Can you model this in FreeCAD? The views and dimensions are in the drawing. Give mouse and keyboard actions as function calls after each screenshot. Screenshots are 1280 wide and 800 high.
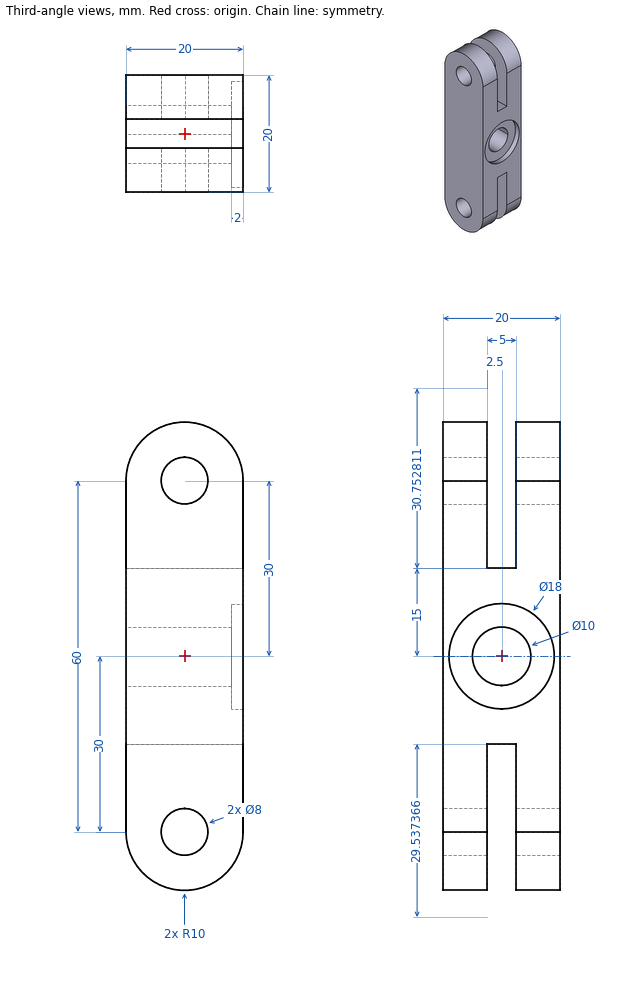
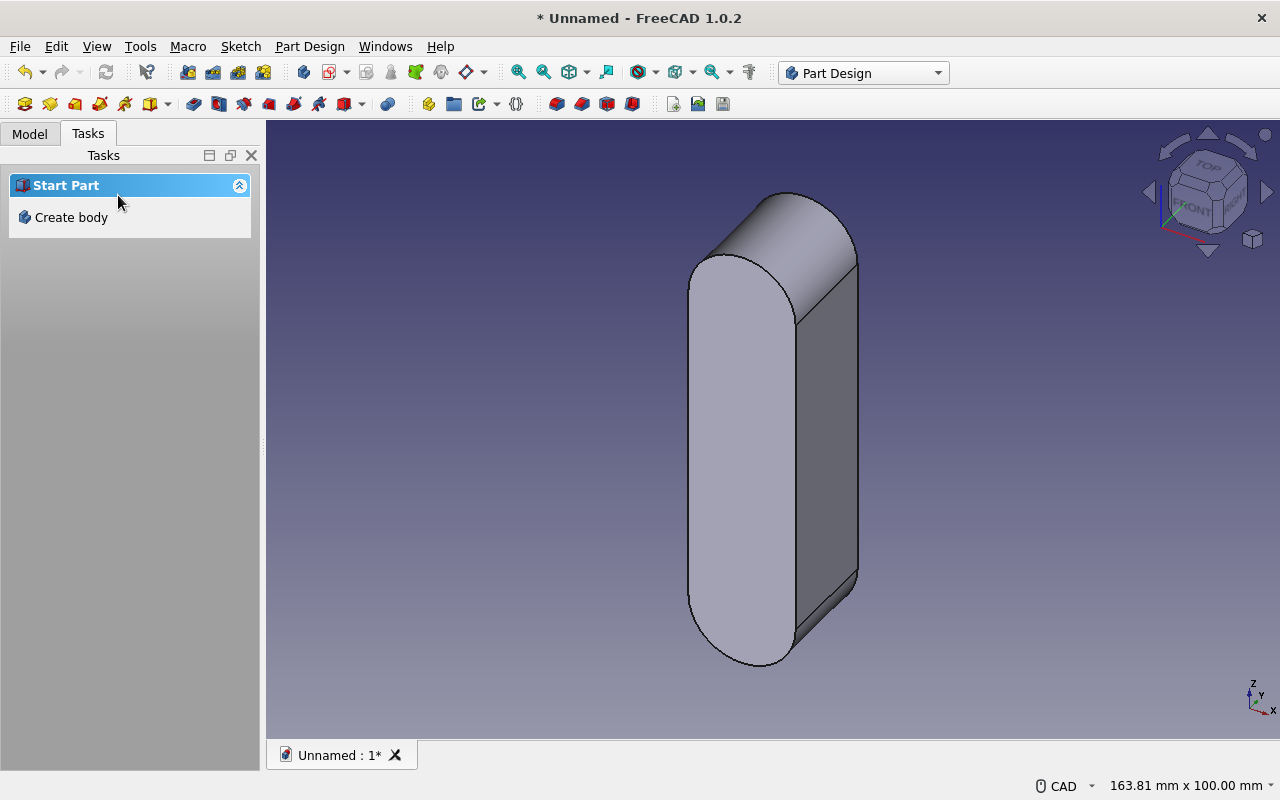
click(328, 72)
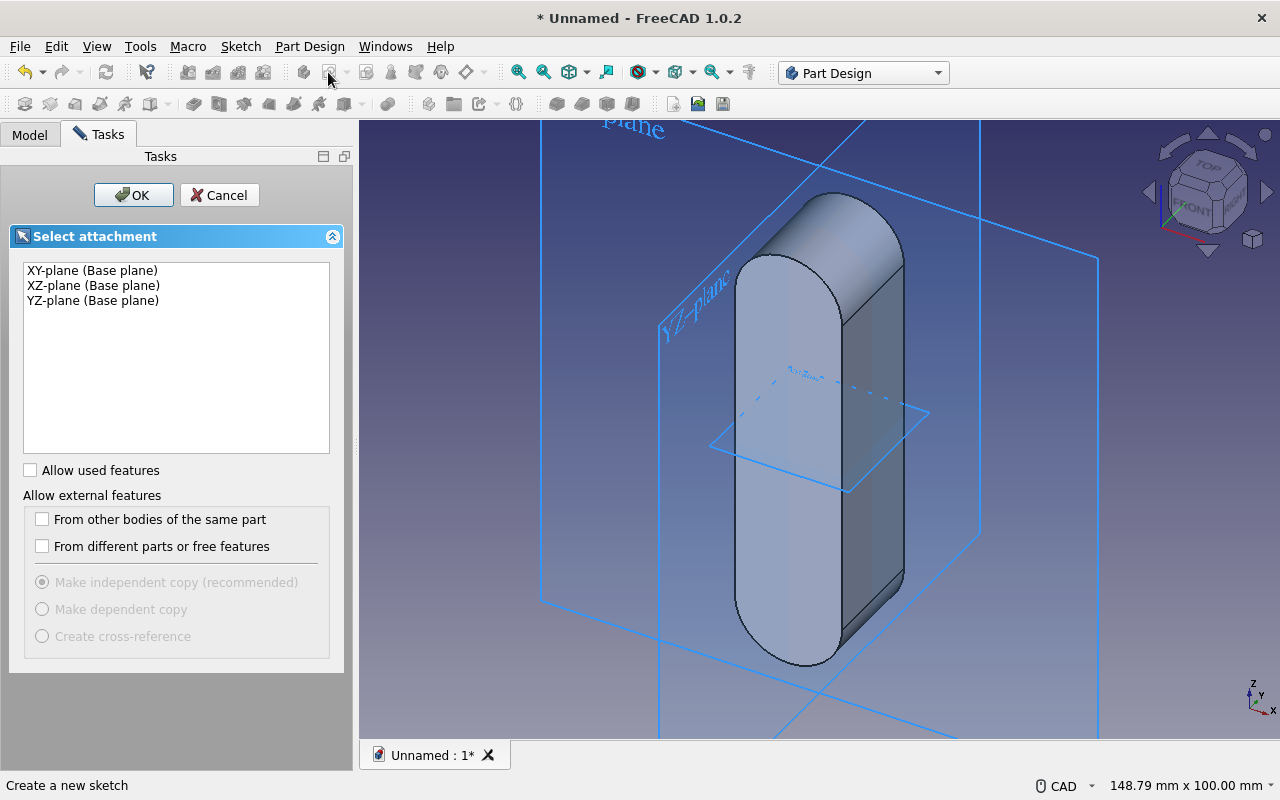
click(84, 286)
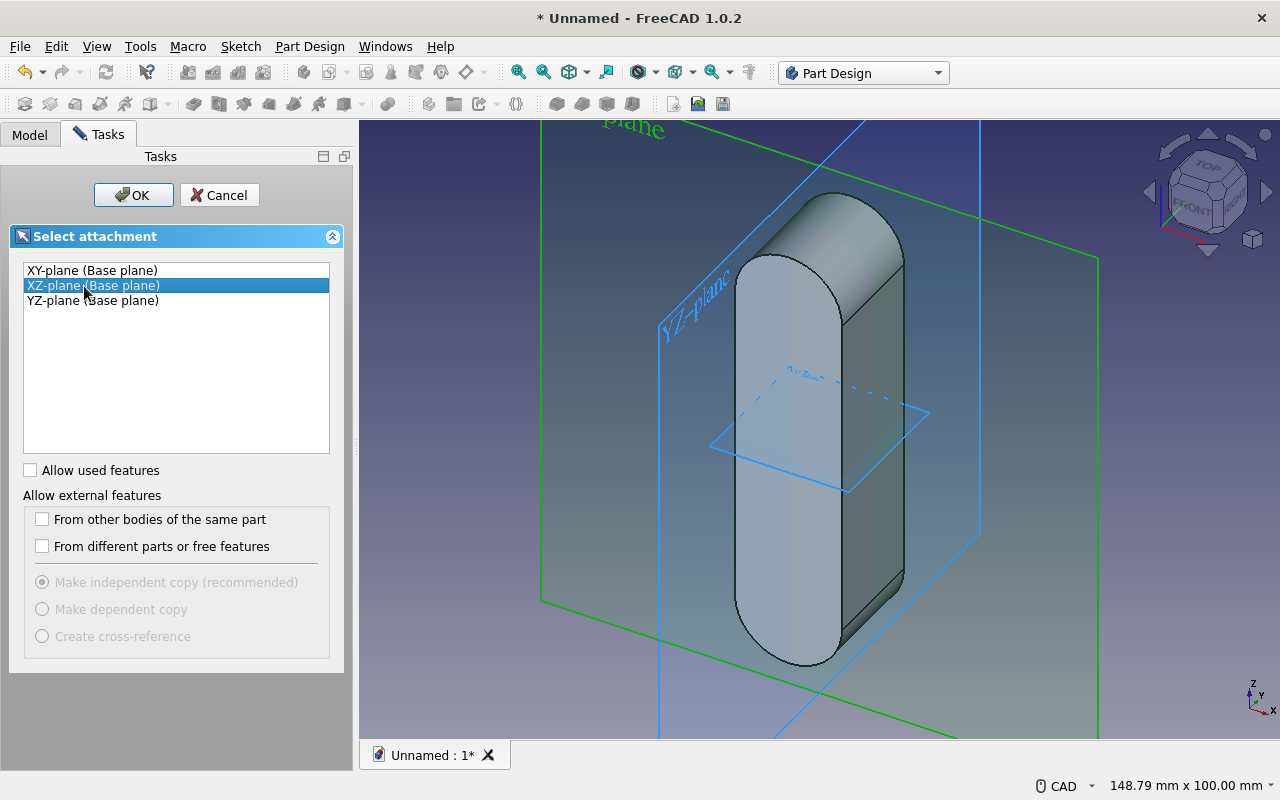
click(134, 195)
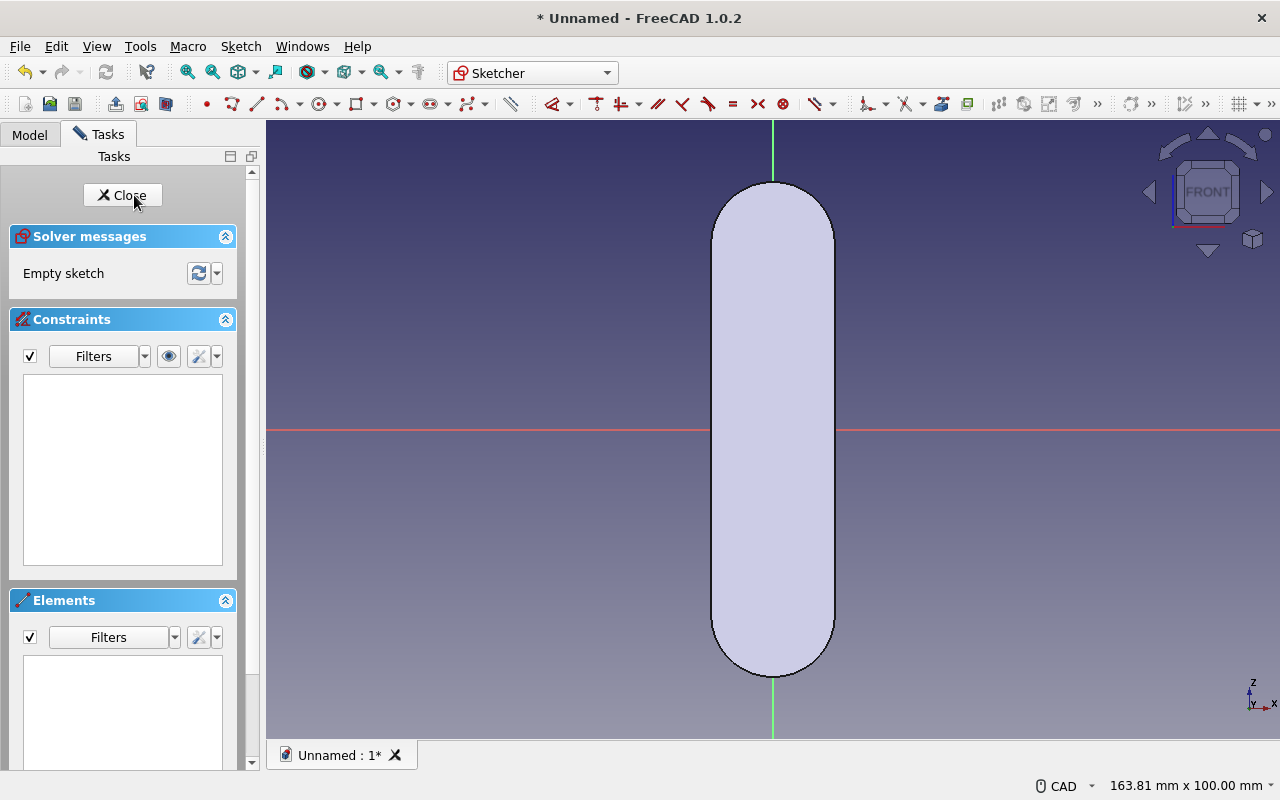
click(166, 104)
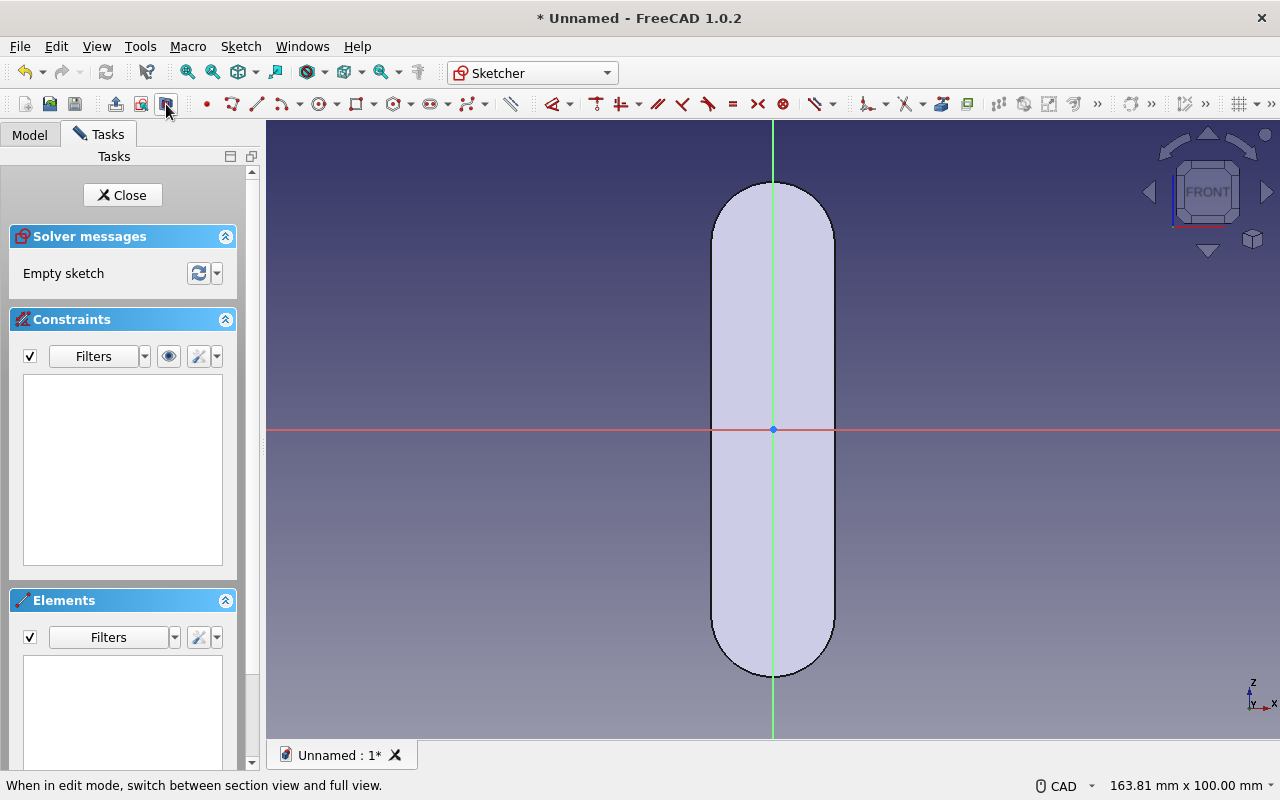
key(g)
key(c)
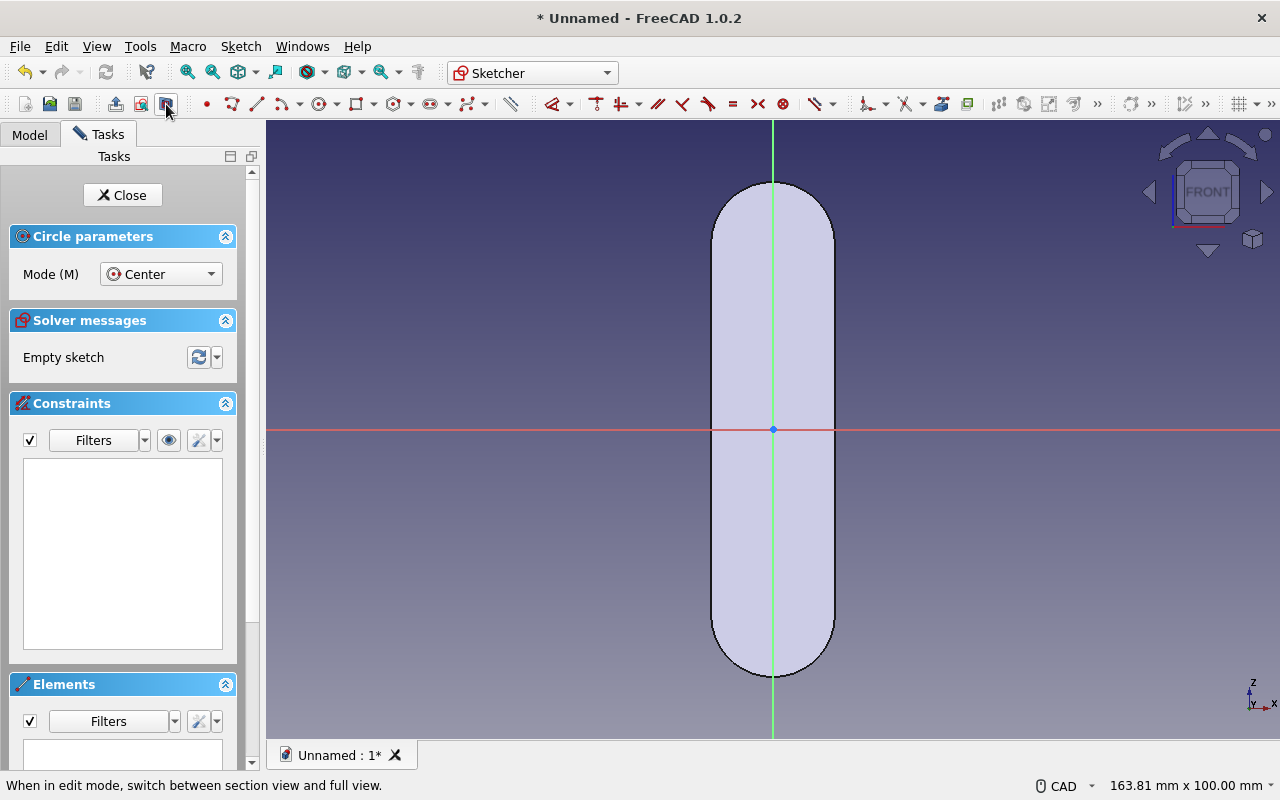
click(773, 615)
click(791, 598)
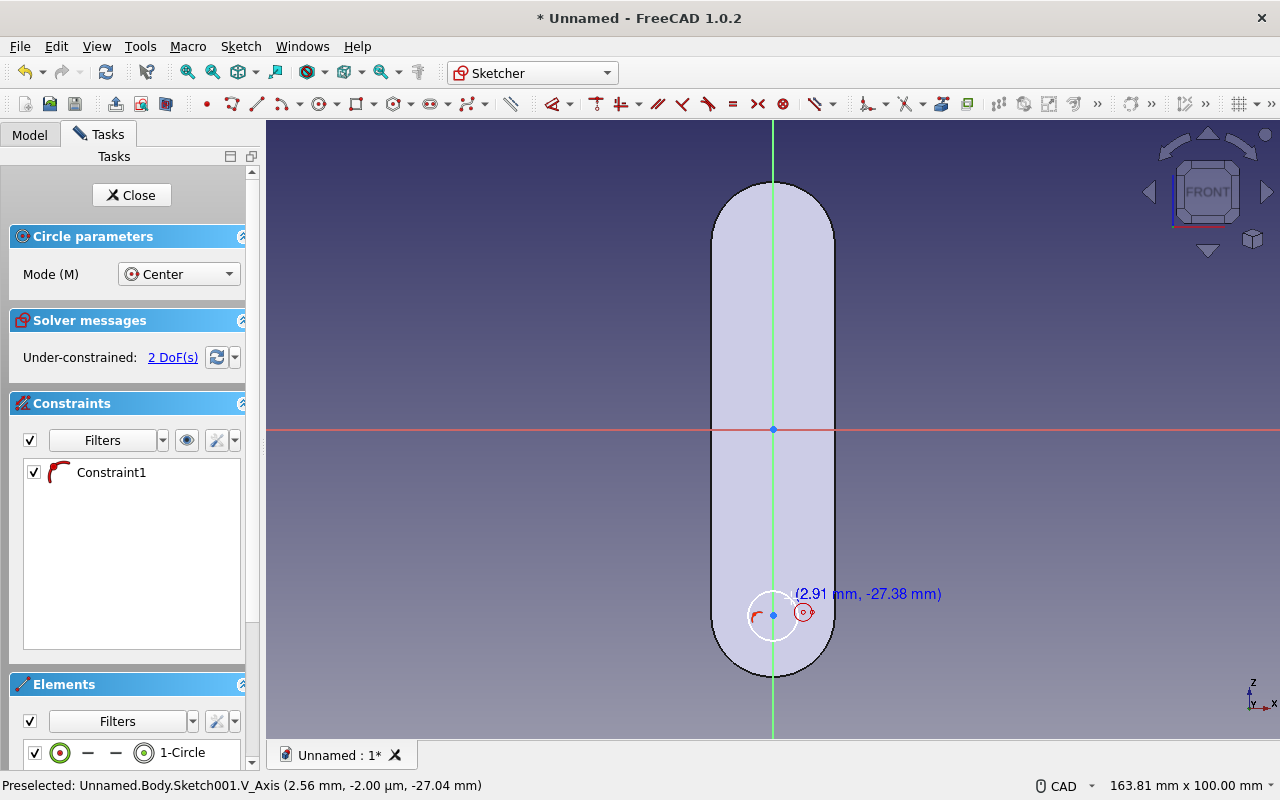
click(773, 244)
click(791, 226)
key(Escape)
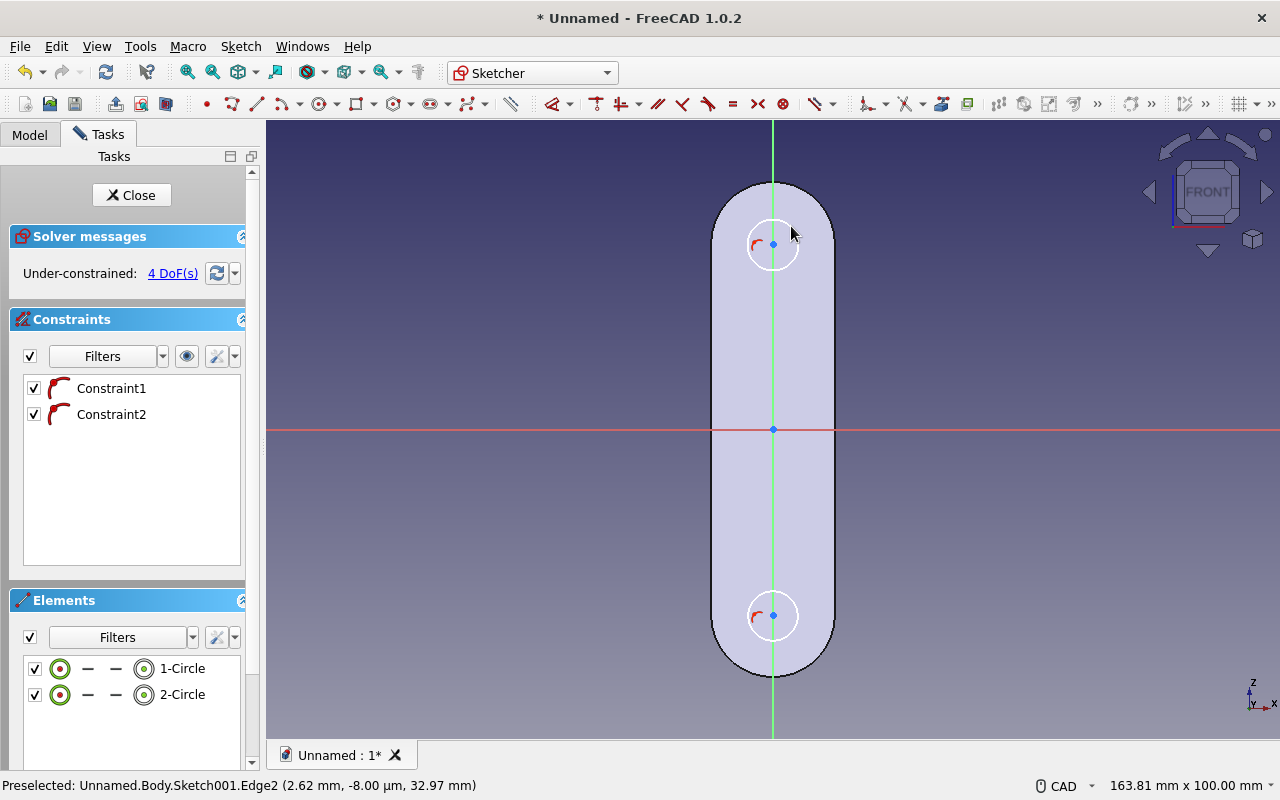
click(790, 598)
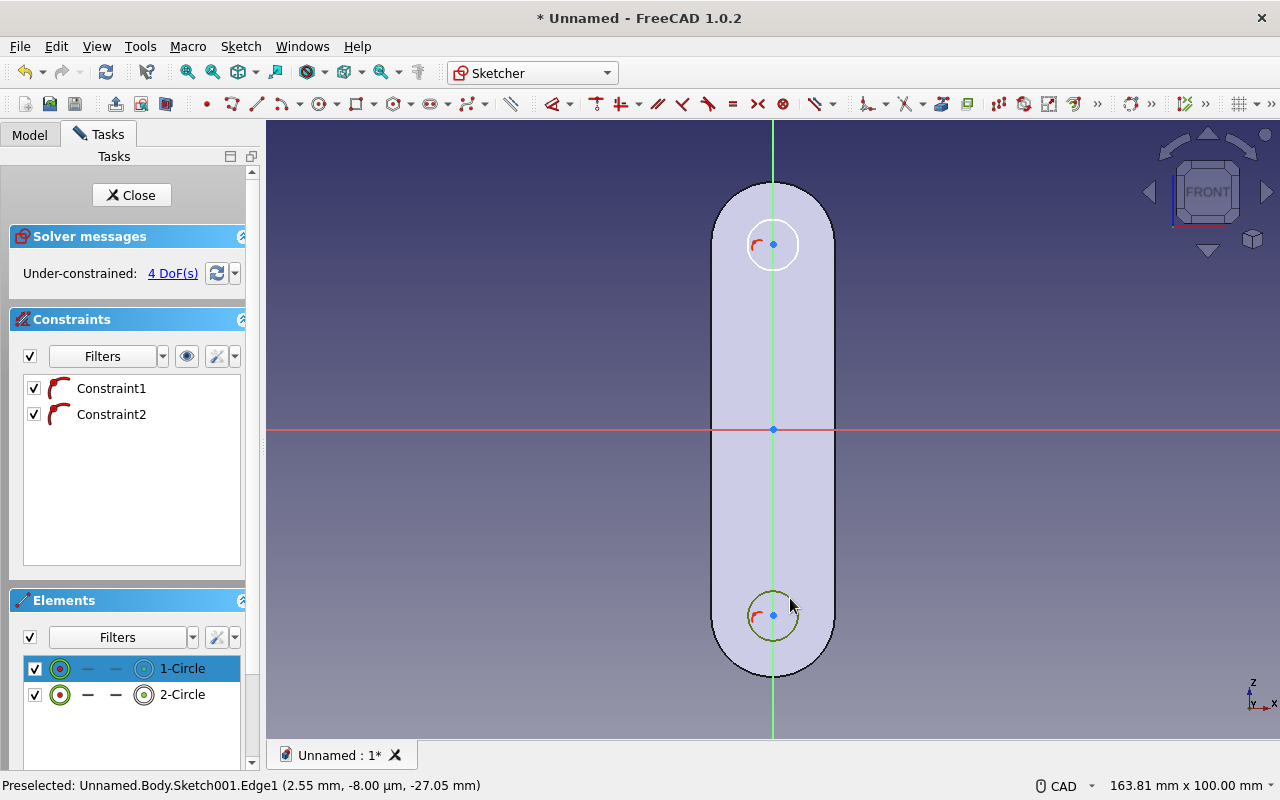
click(791, 227)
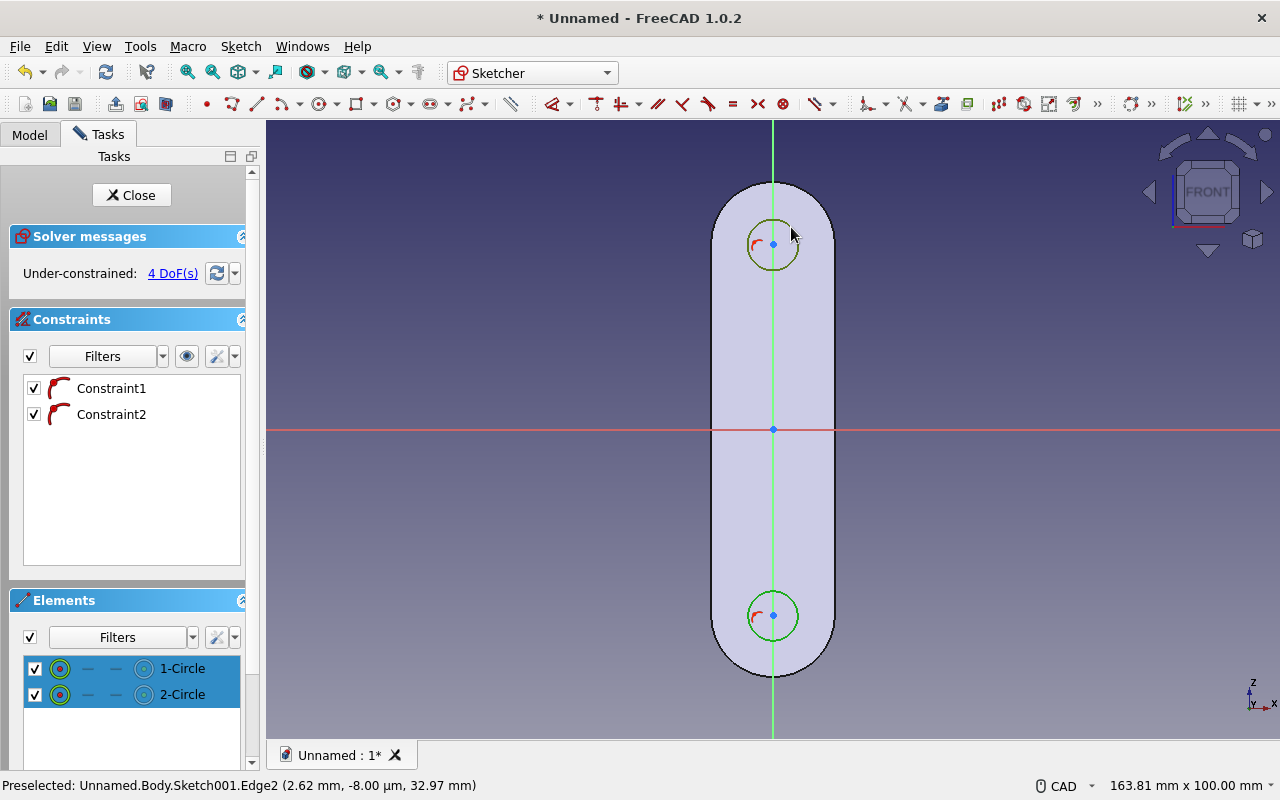
click(733, 104)